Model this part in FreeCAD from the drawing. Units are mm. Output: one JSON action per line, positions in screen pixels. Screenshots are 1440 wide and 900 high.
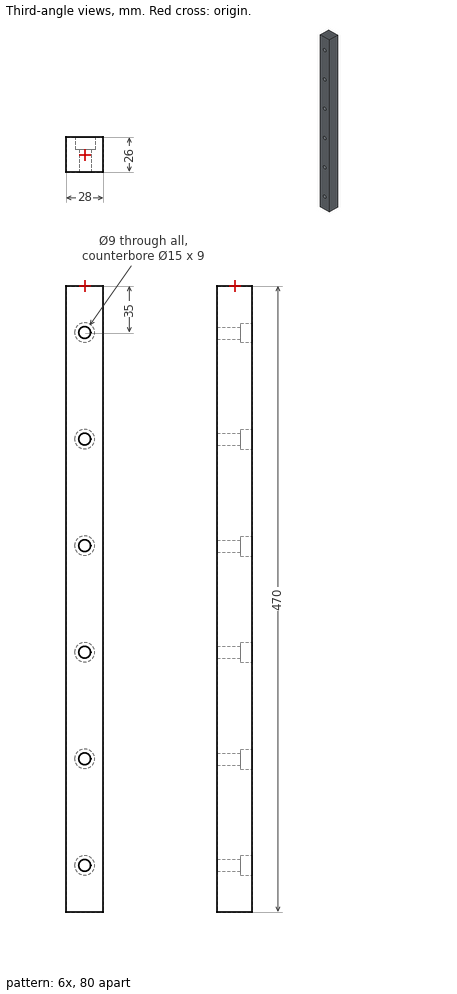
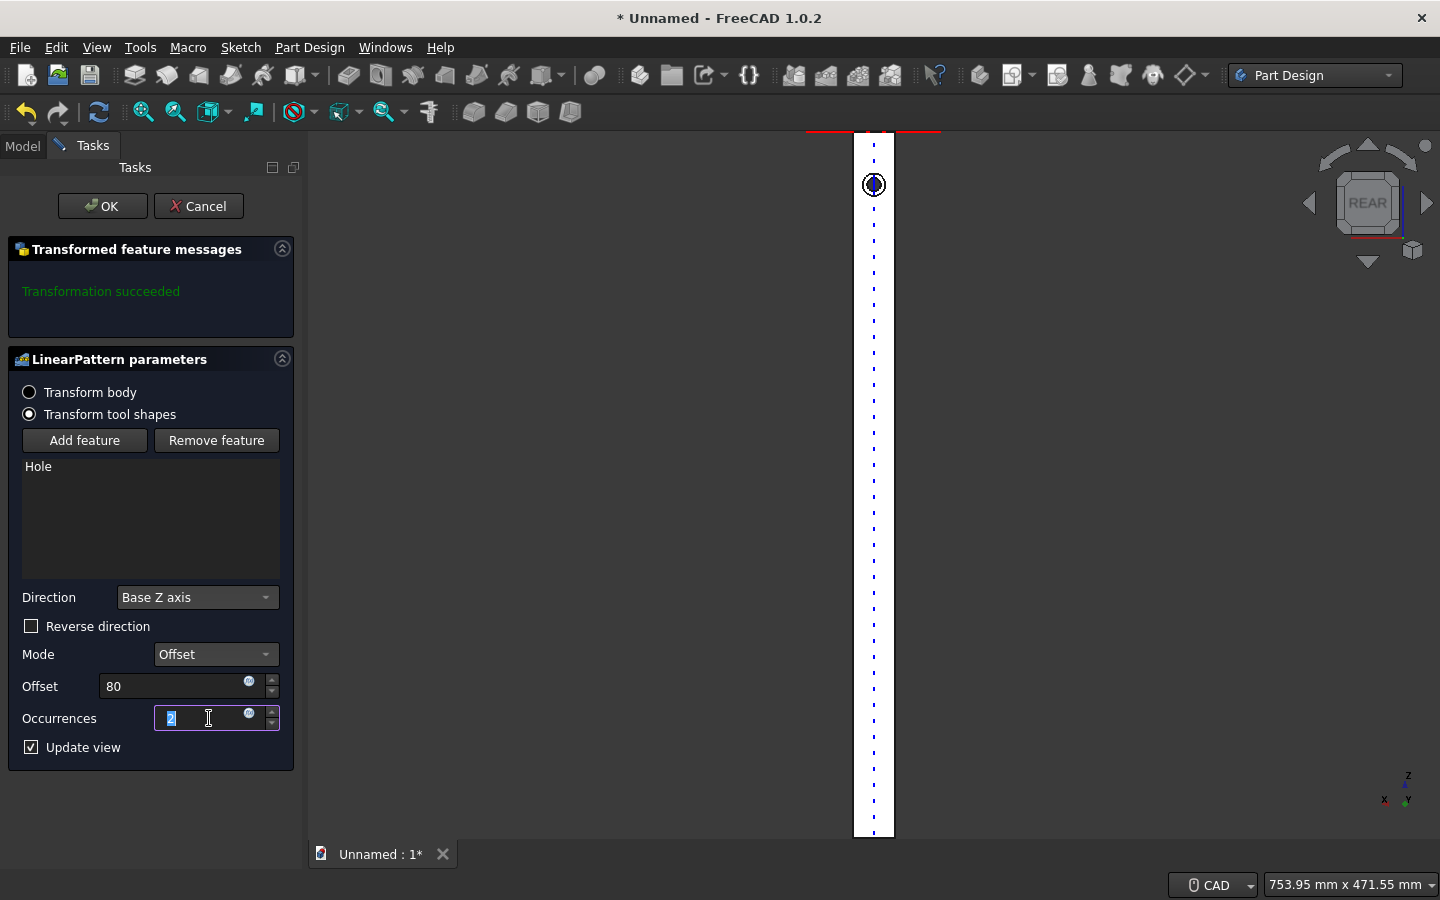
{"action": "type", "text": "6"}
{"action": "key", "text": "Tab"}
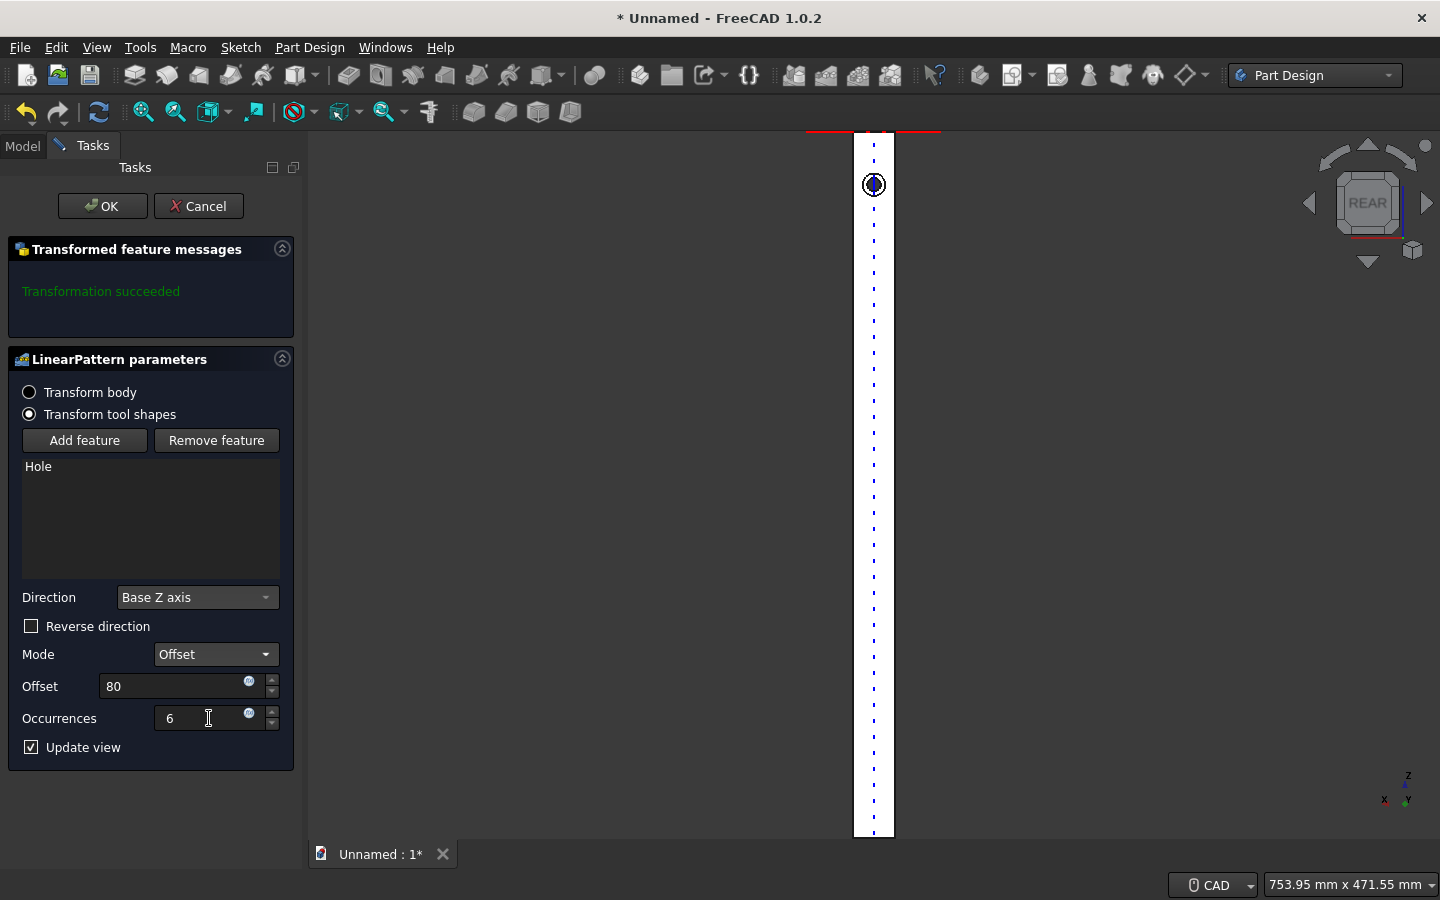
{"action": "left_click", "coordinate": [30, 626]}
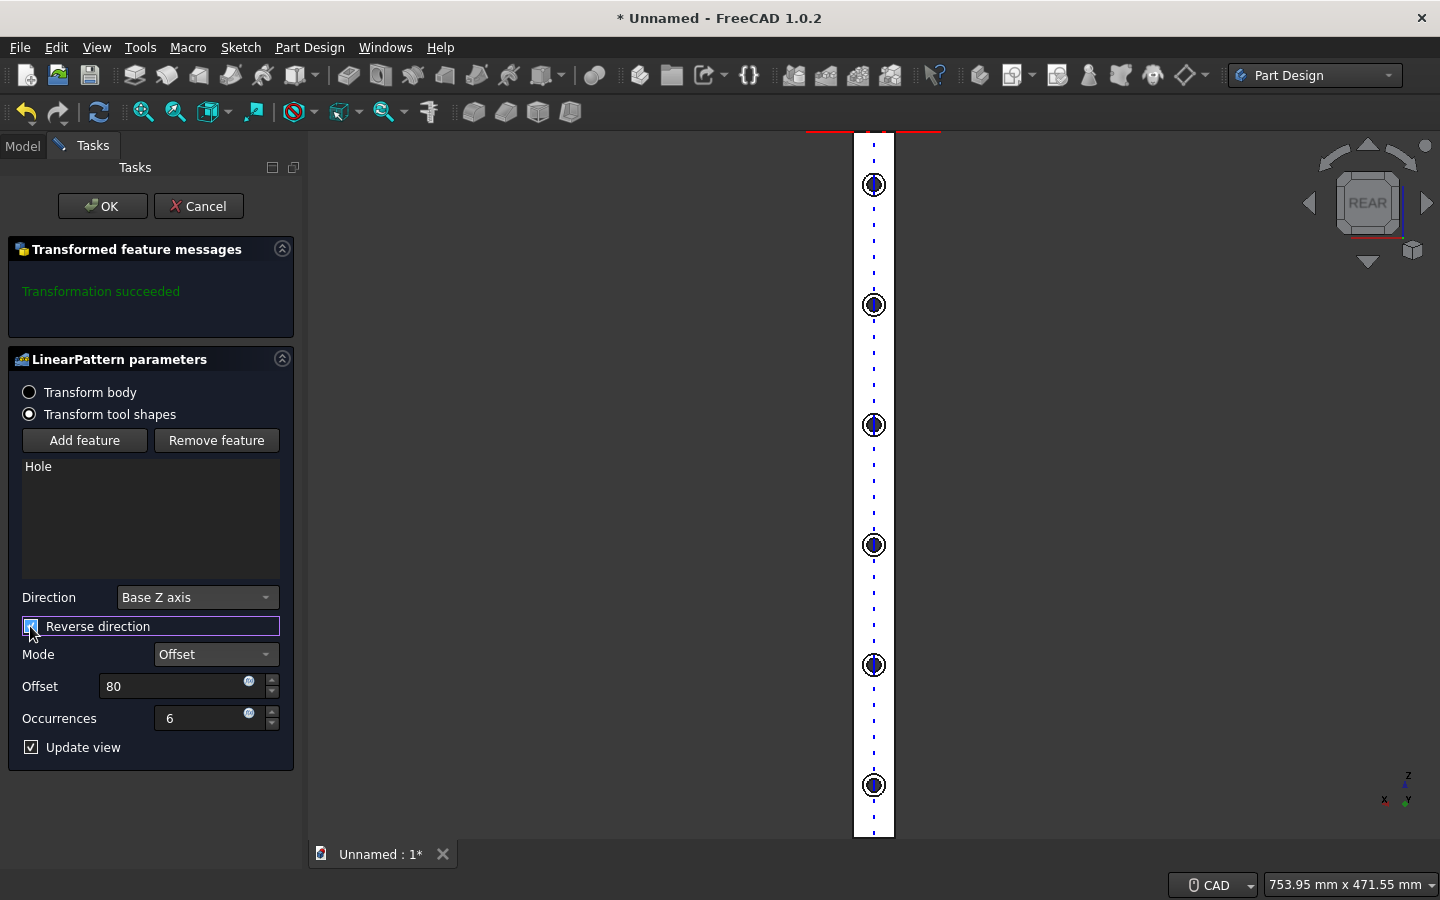
{"action": "left_click", "coordinate": [103, 206]}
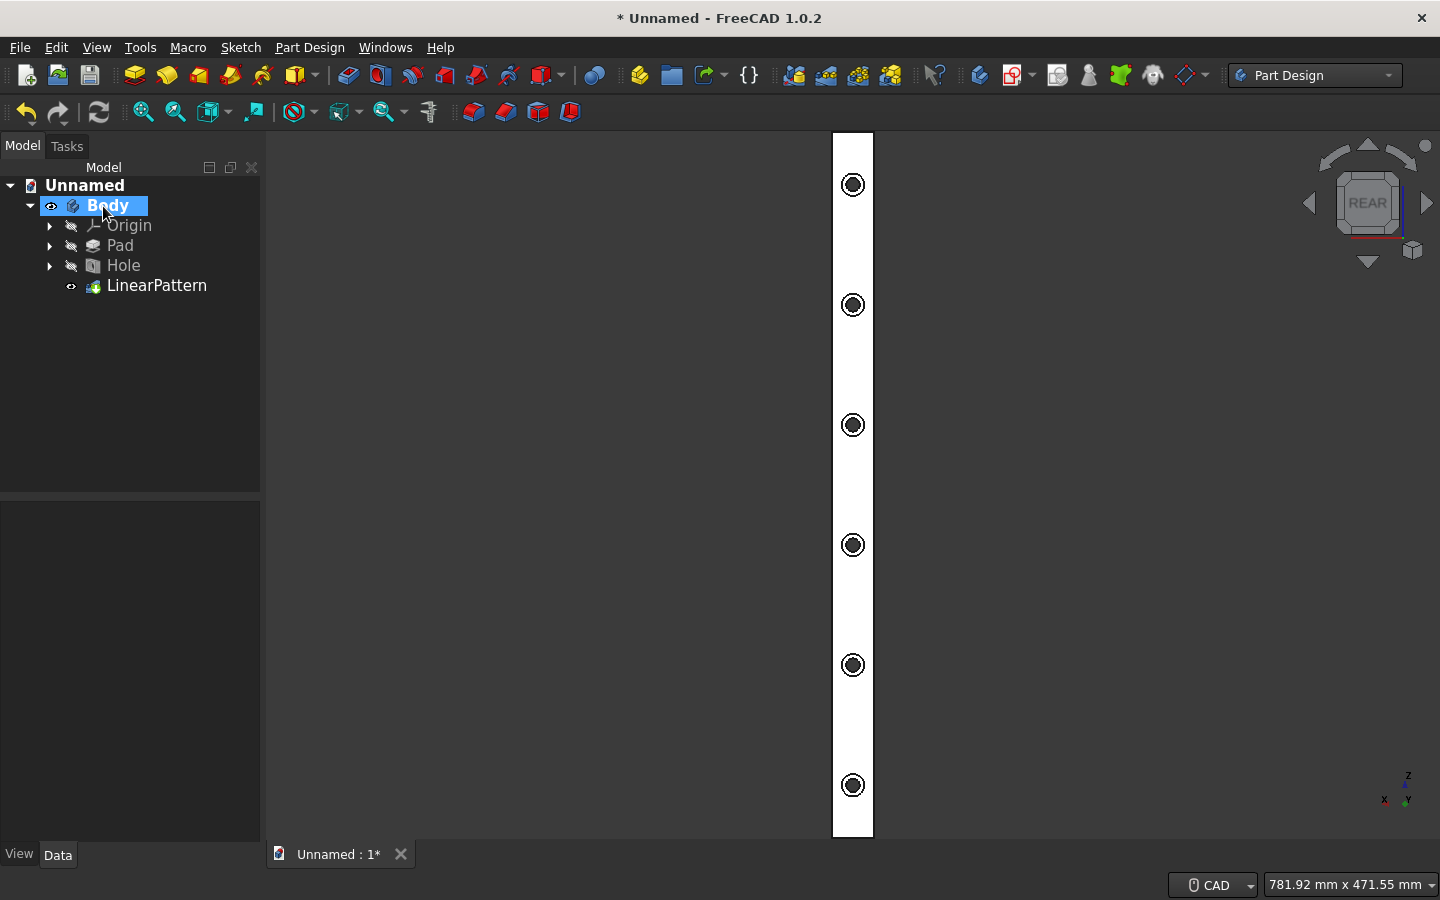
{"action": "key", "text": "0"}